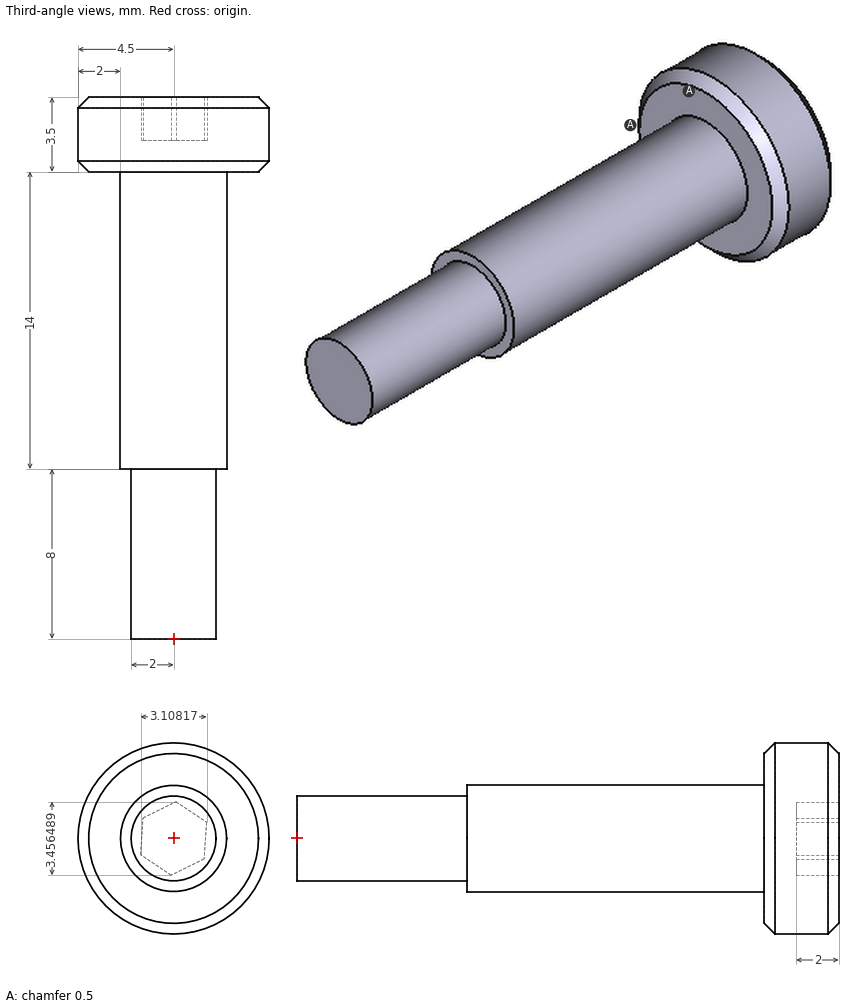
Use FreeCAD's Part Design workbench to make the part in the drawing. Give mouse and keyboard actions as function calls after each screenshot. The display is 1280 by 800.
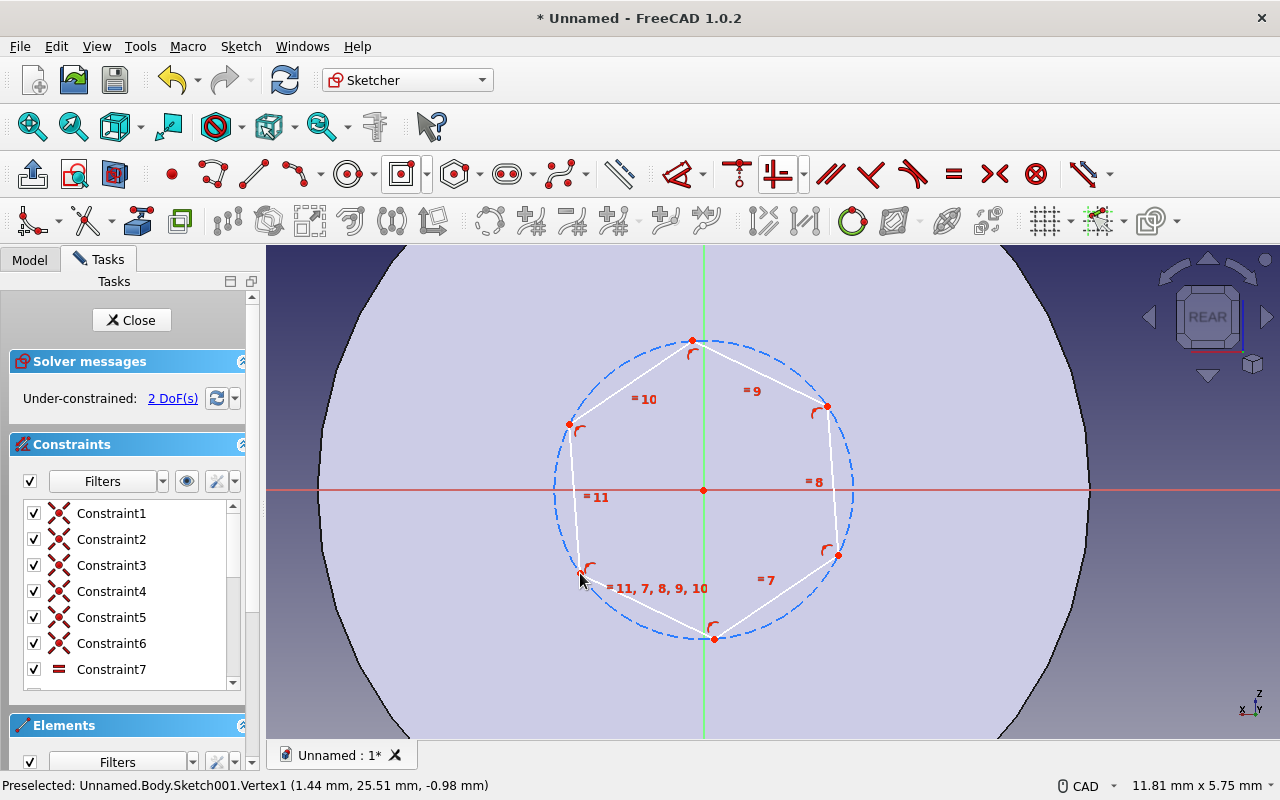
click(676, 174)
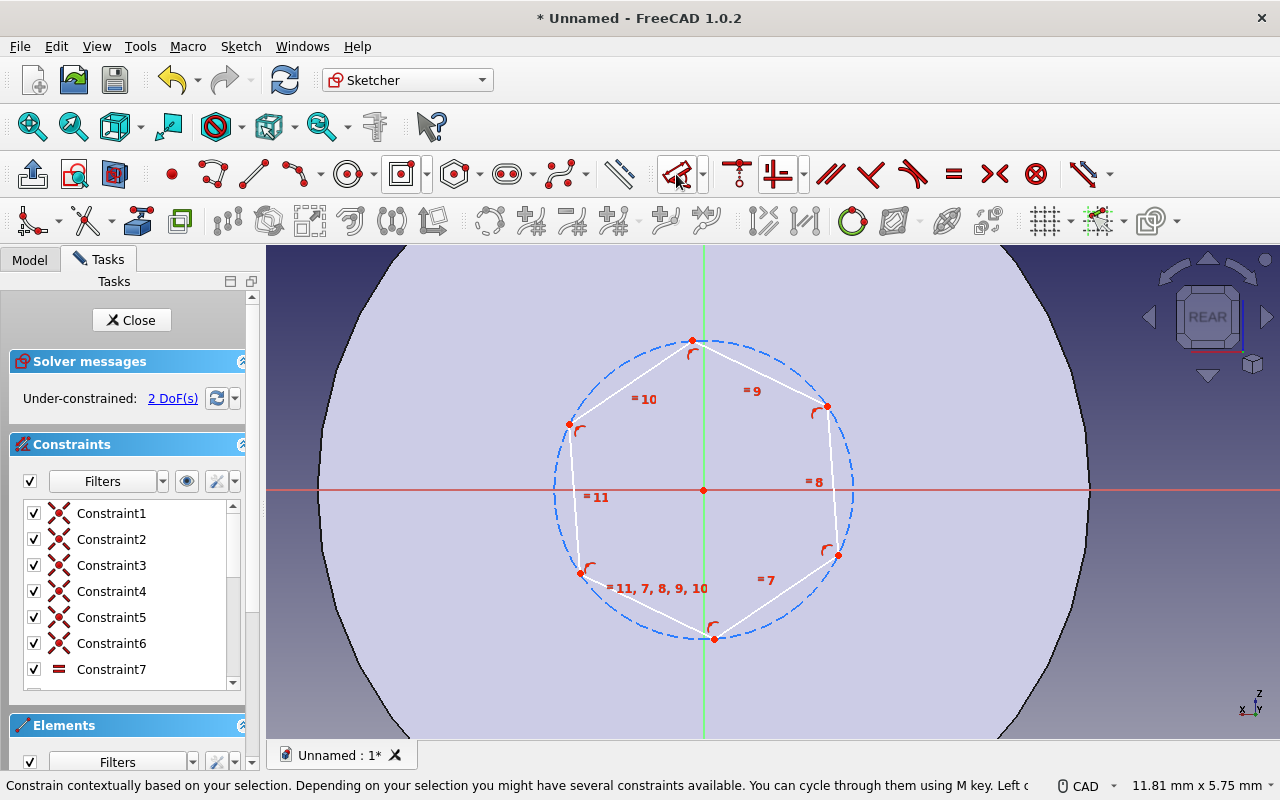
click(569, 425)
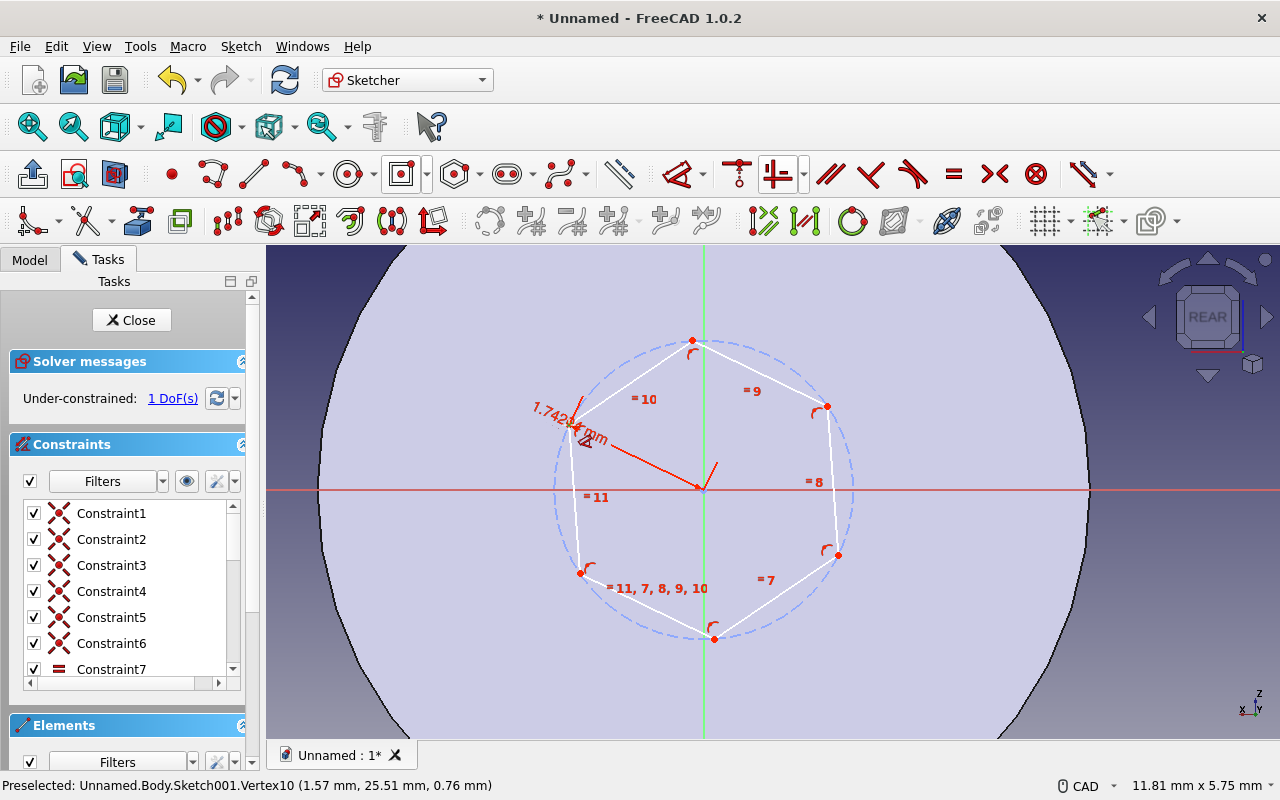
click(838, 555)
click(766, 391)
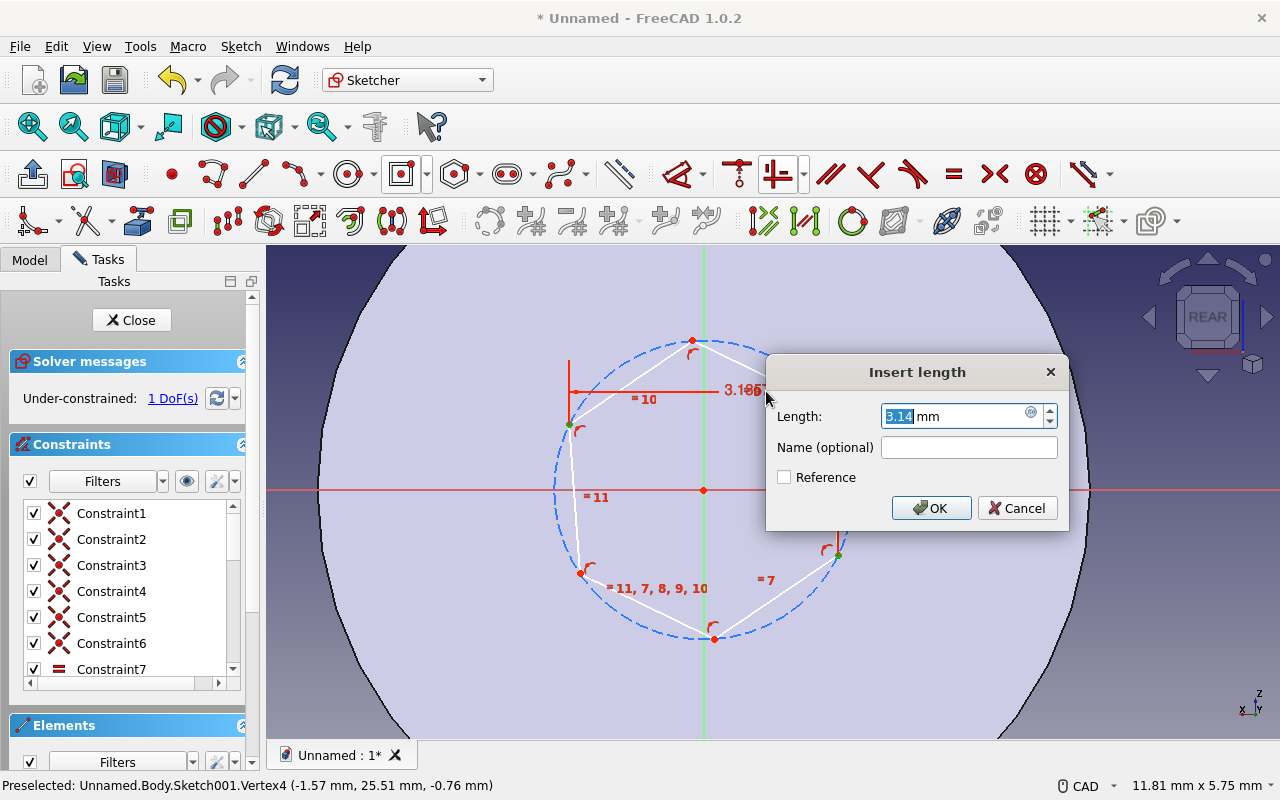
text(3.10817)
key(Return)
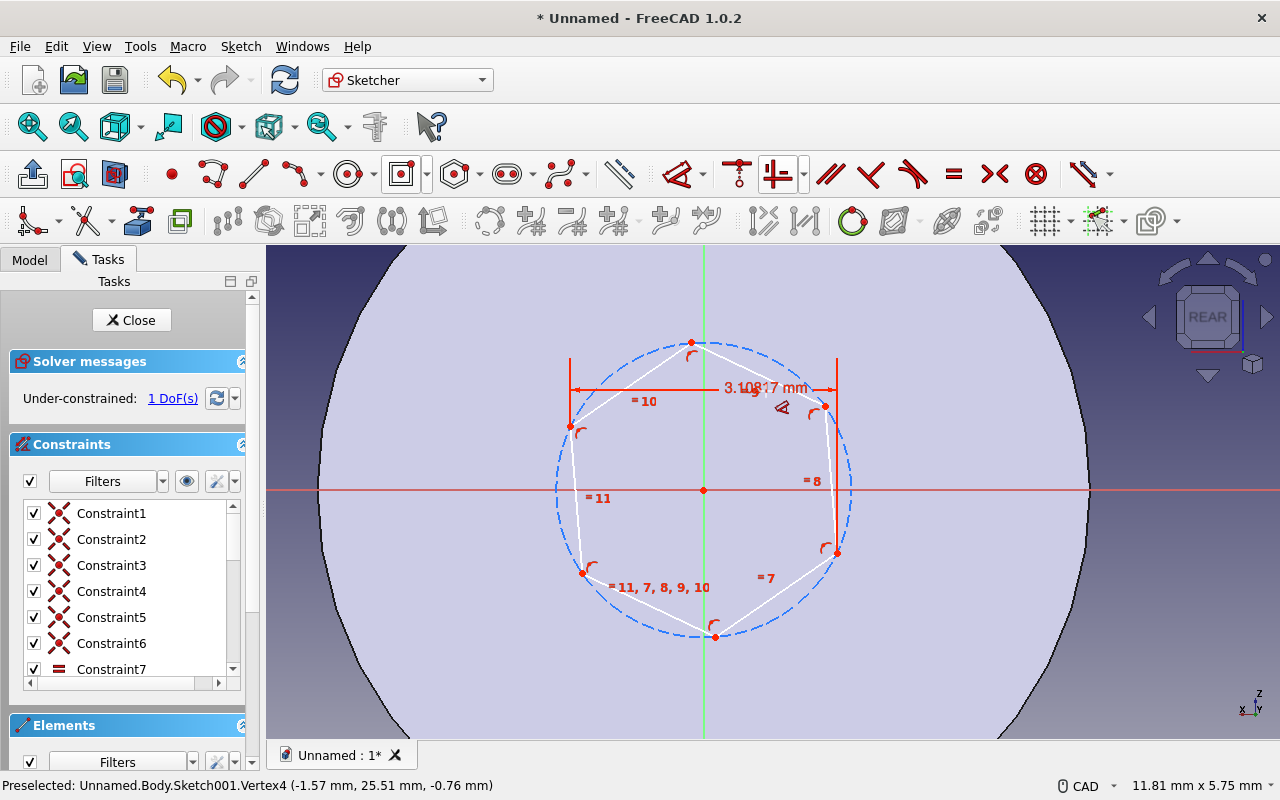
click(716, 637)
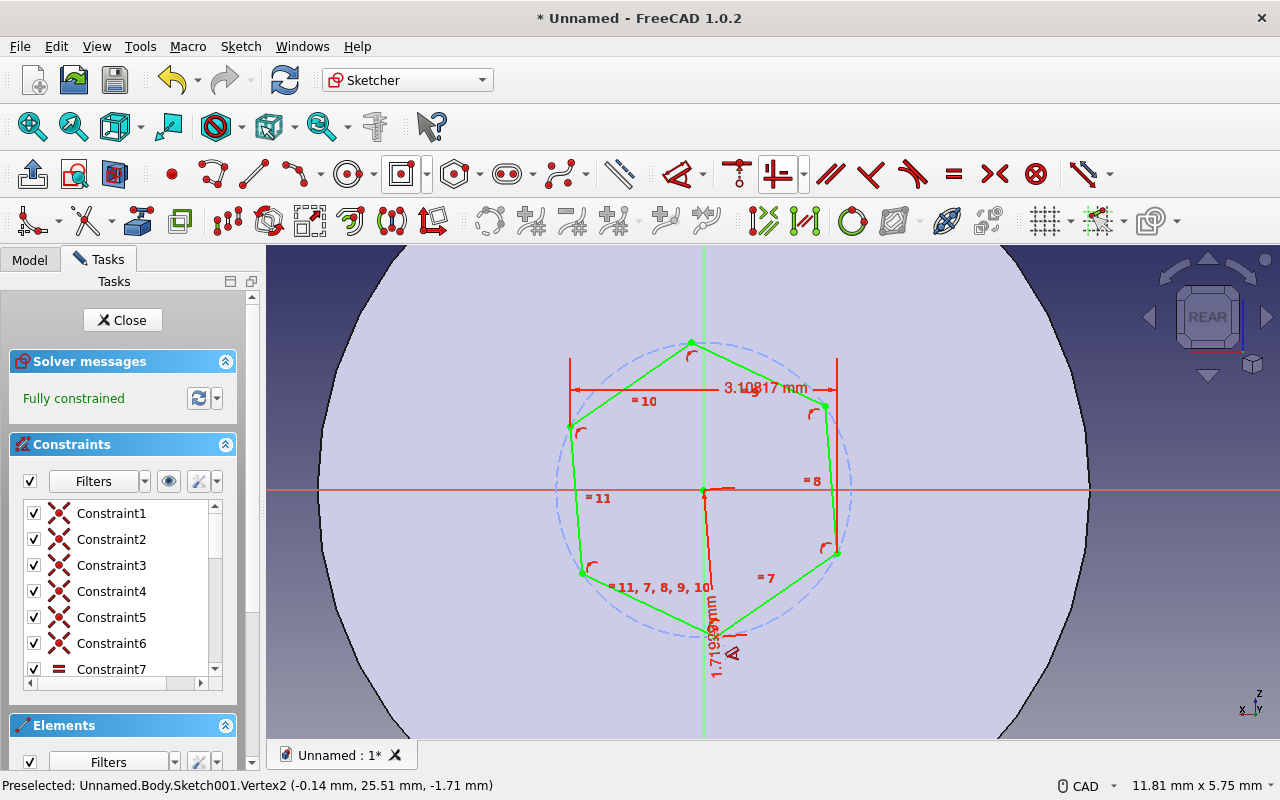
click(692, 343)
click(750, 422)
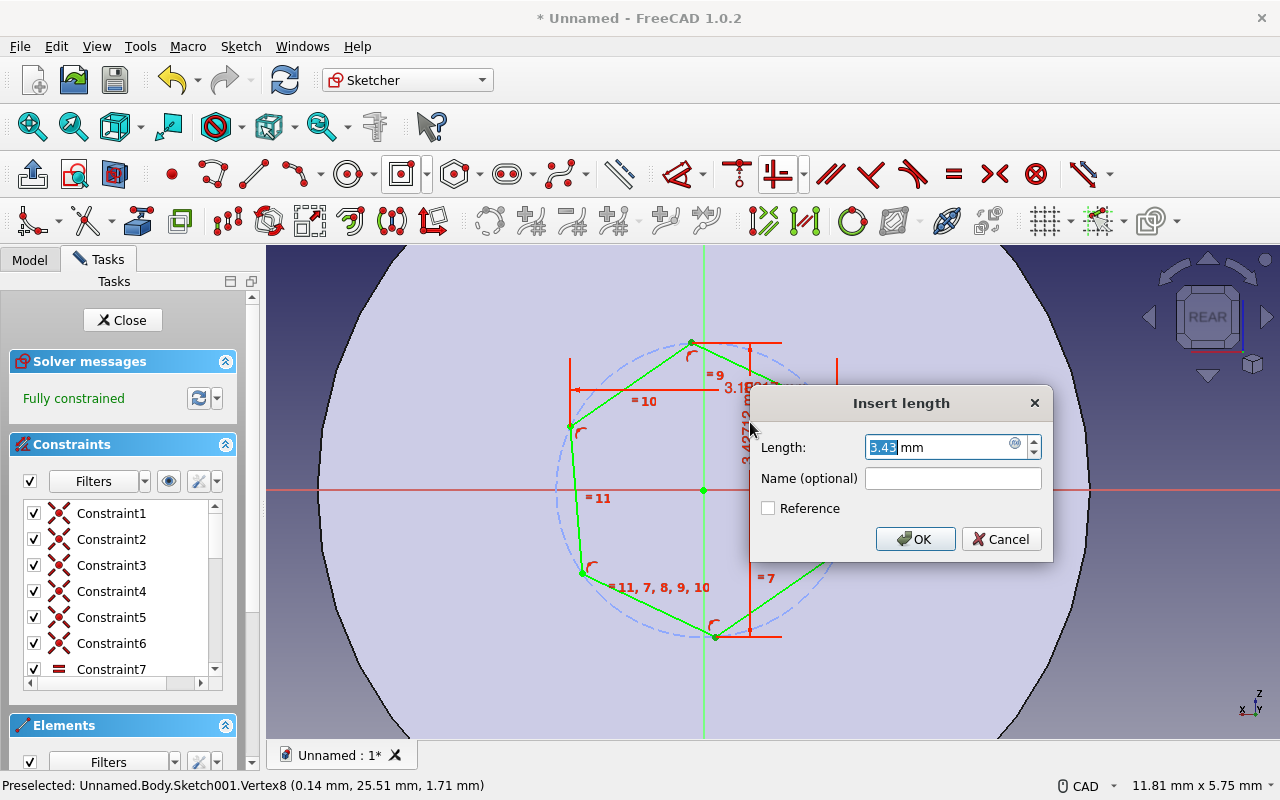
text(3.456489)
key(Return)
key(Escape)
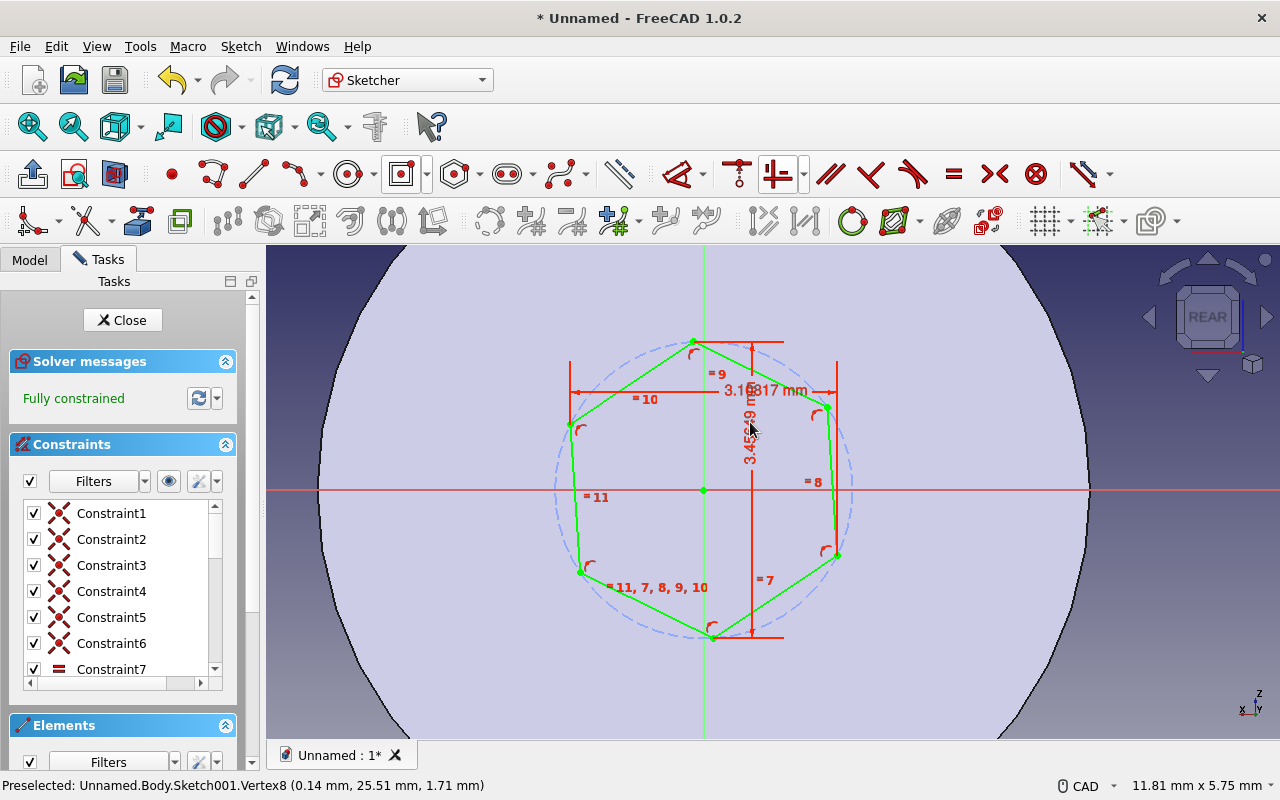
click(123, 320)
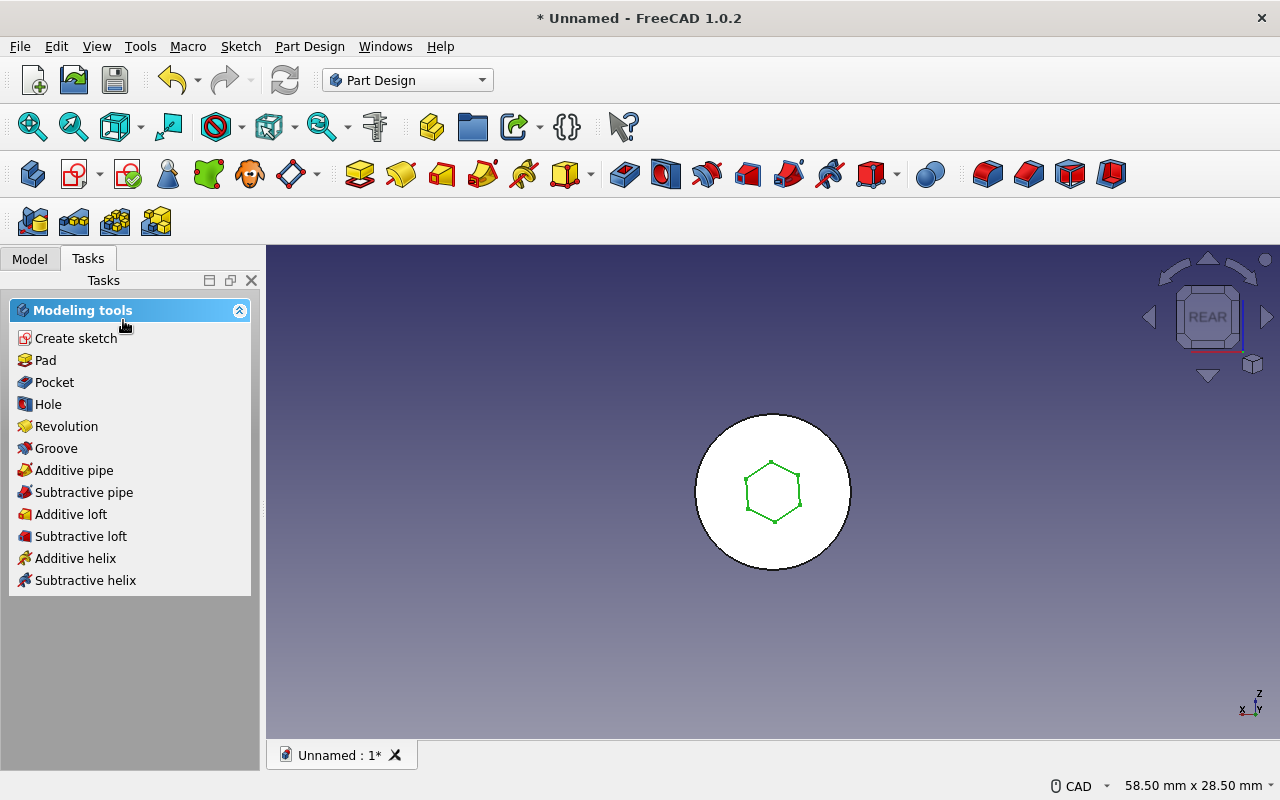
click(625, 174)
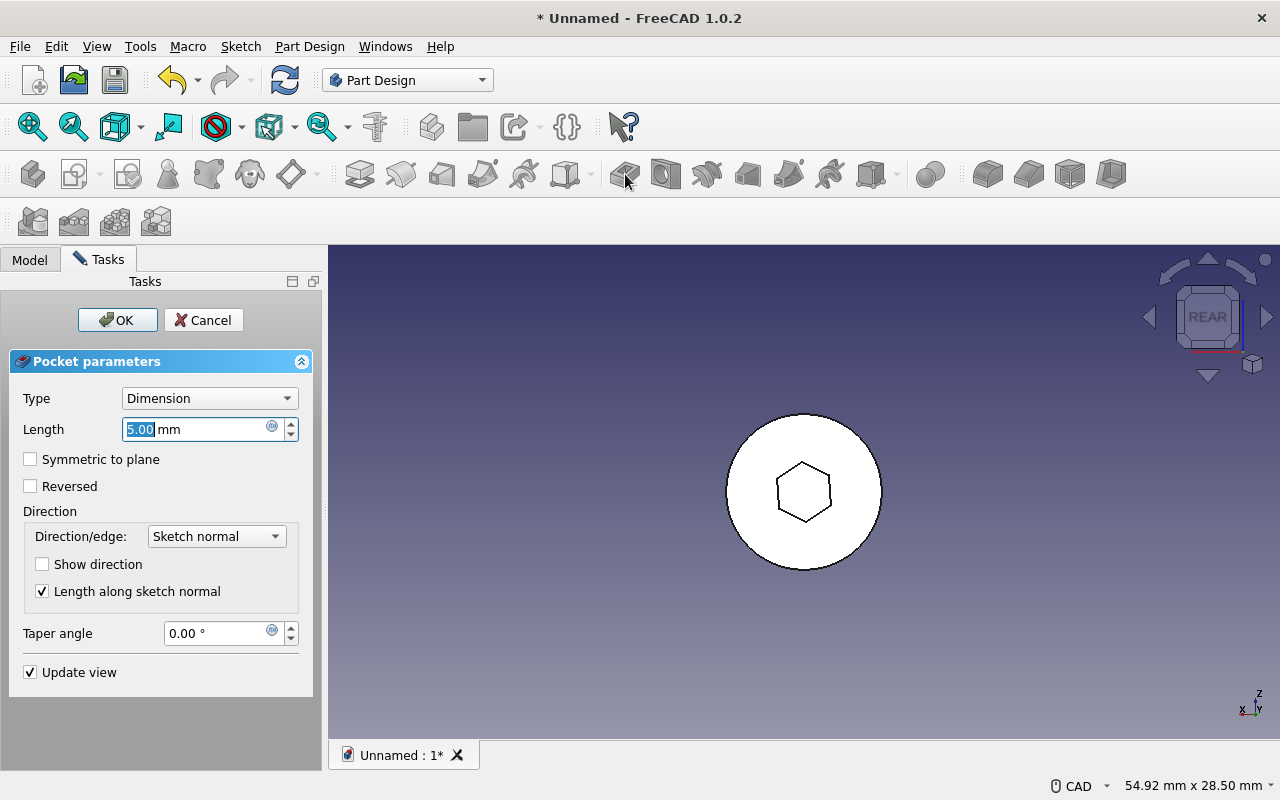
text(2)
key(Tab)